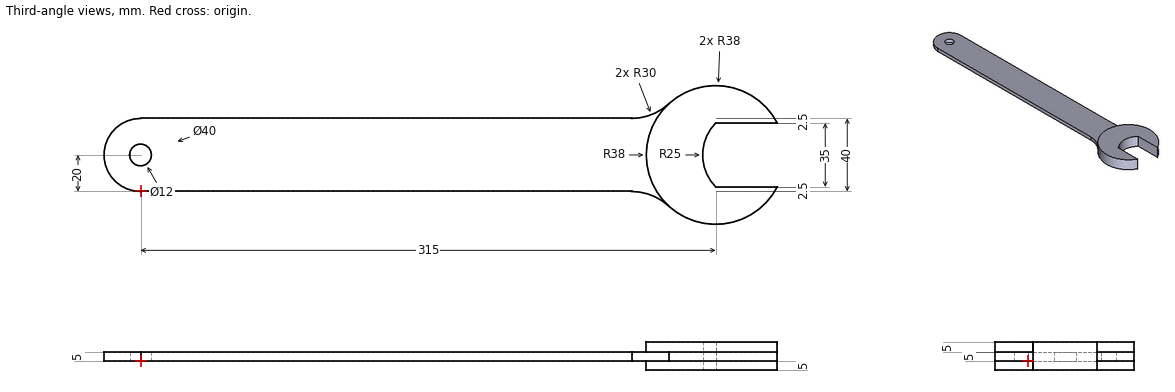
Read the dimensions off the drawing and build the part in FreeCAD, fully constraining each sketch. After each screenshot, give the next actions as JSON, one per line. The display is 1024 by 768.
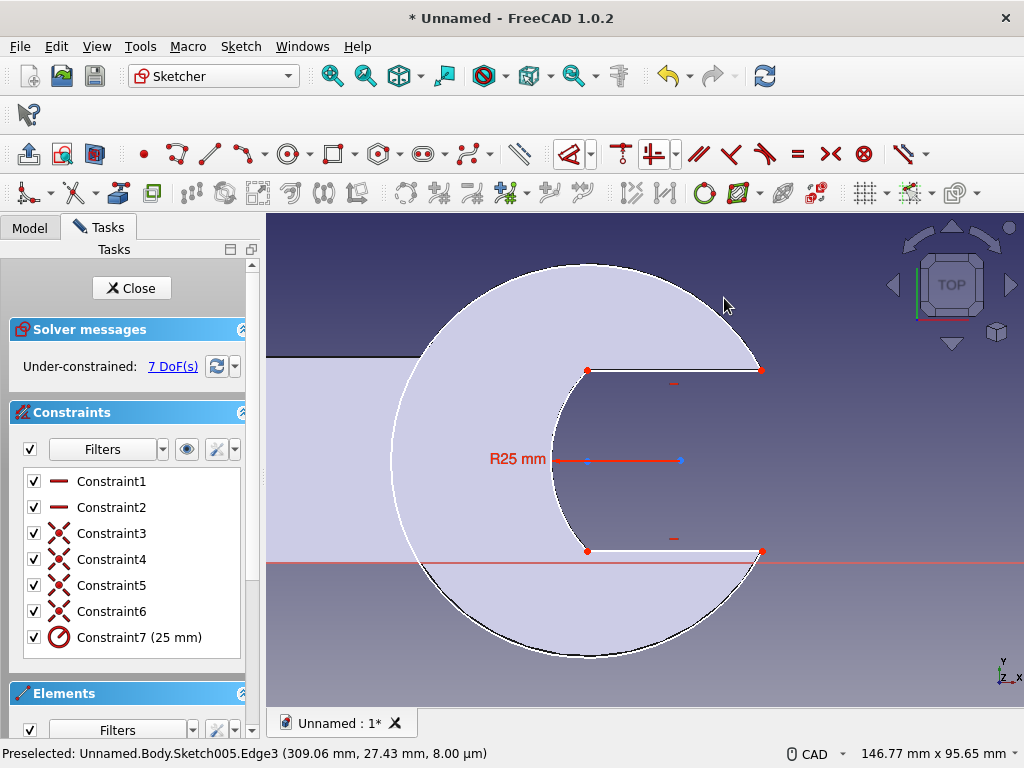
{"action": "left_click", "coordinate": [492, 290]}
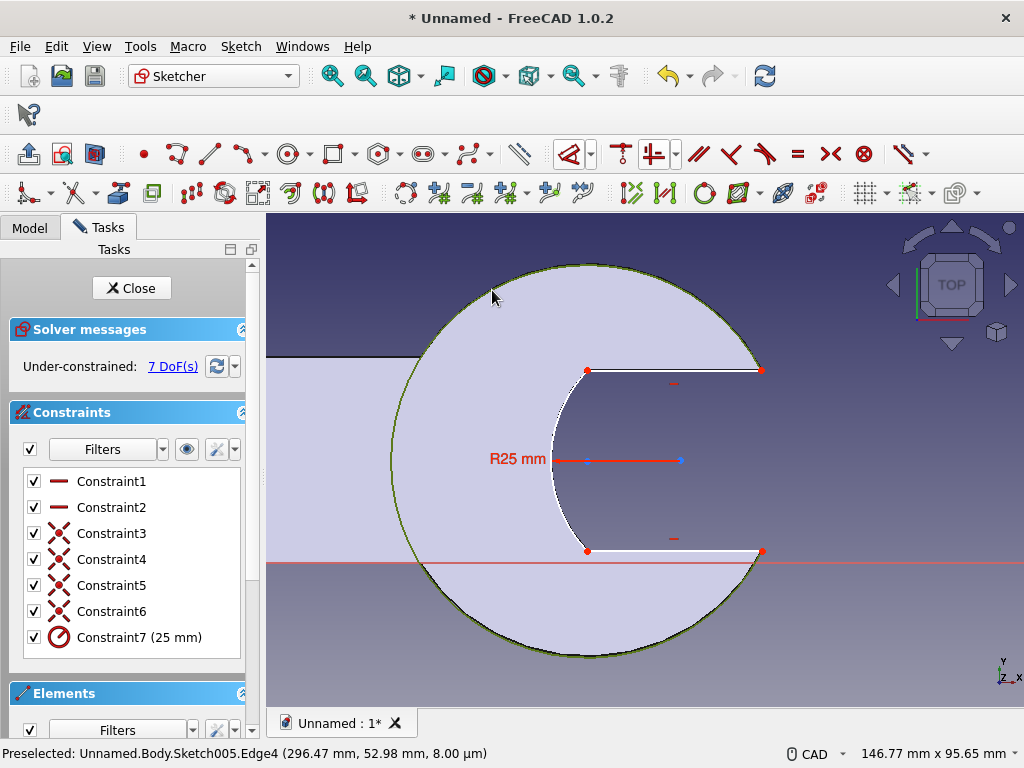
{"action": "left_click", "coordinate": [590, 154]}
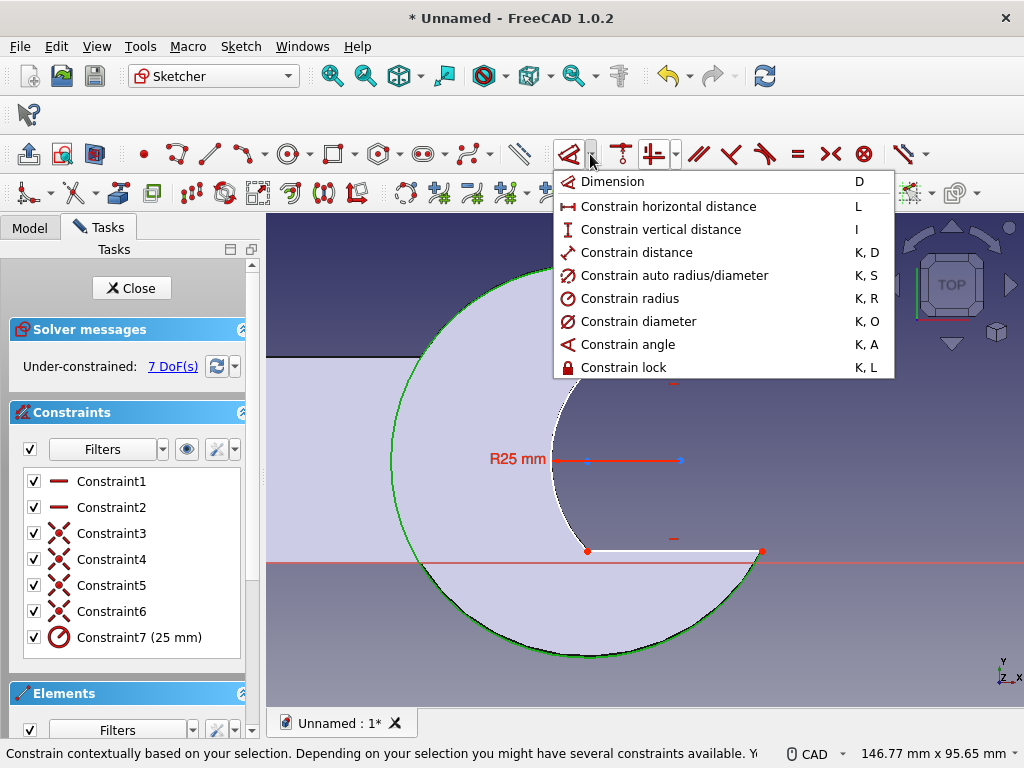
{"action": "left_click", "coordinate": [724, 298]}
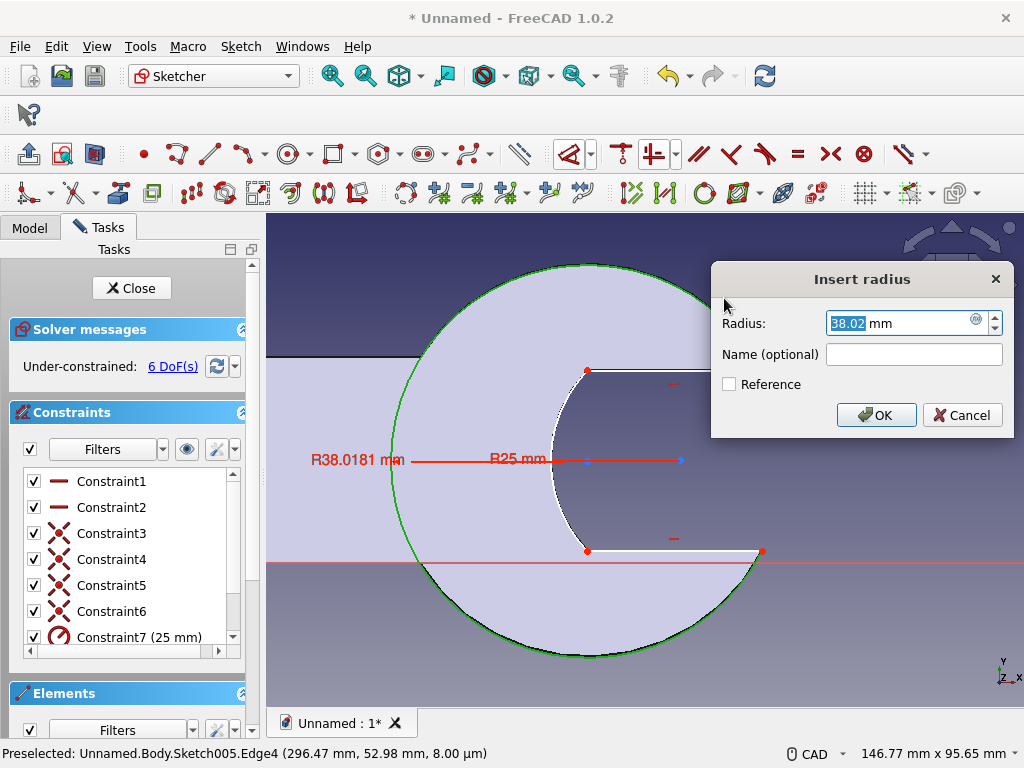
{"action": "type", "text": "38"}
{"action": "key", "text": "Return"}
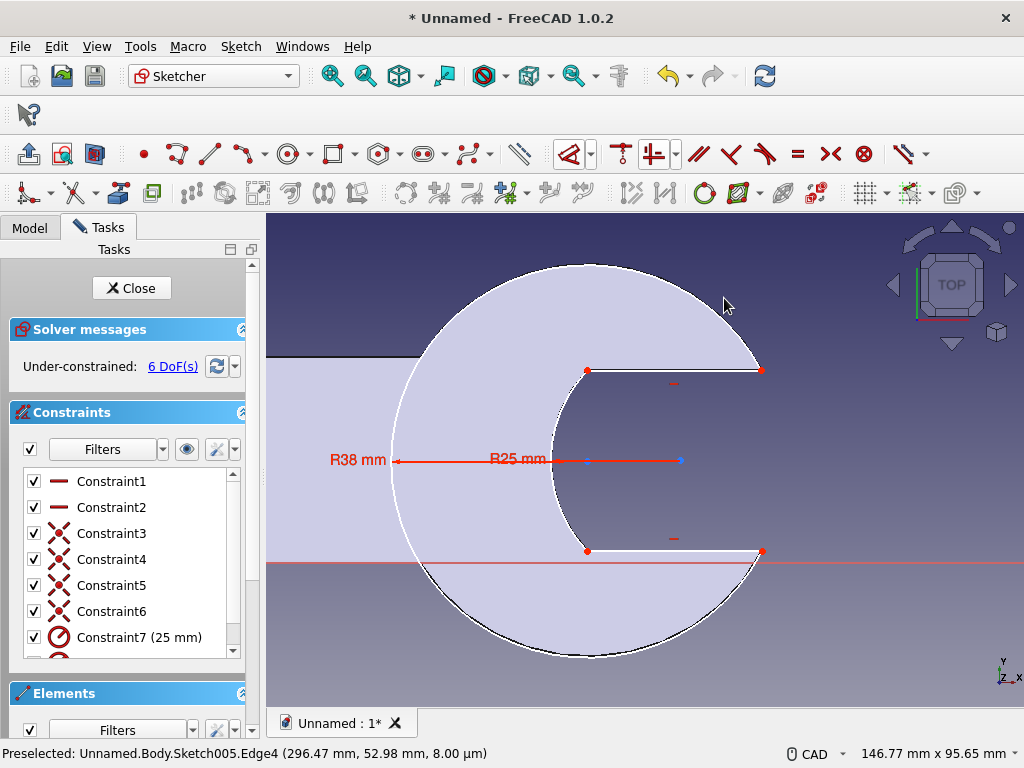
{"action": "left_click", "coordinate": [680, 461]}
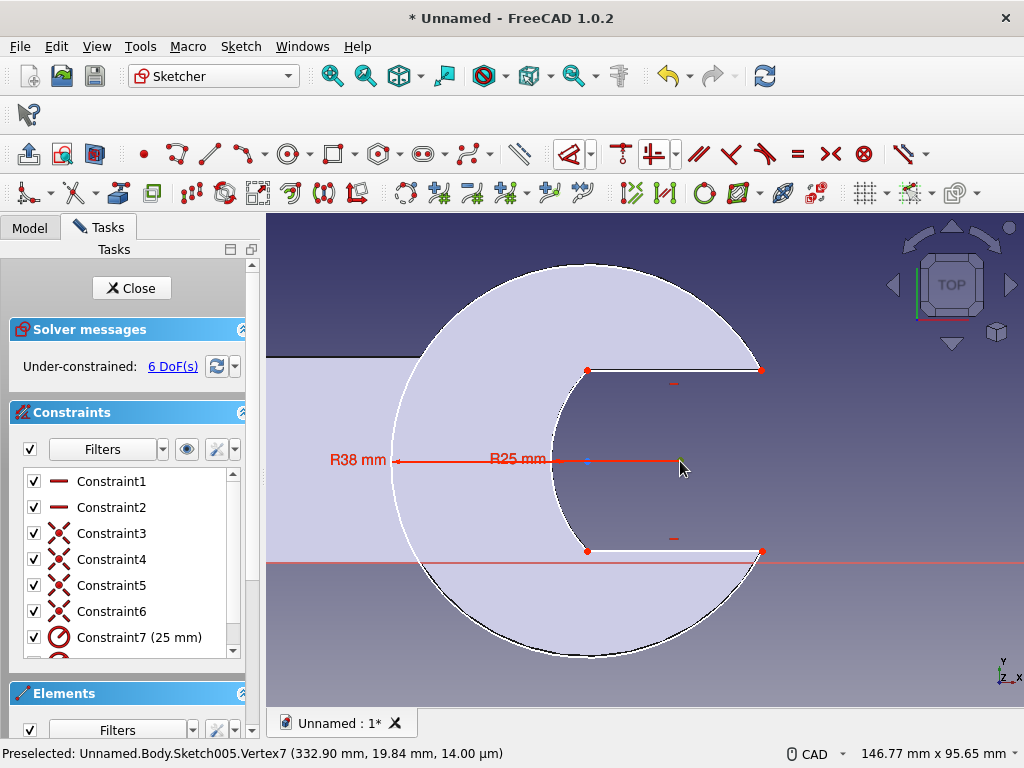
{"action": "left_click", "coordinate": [590, 154]}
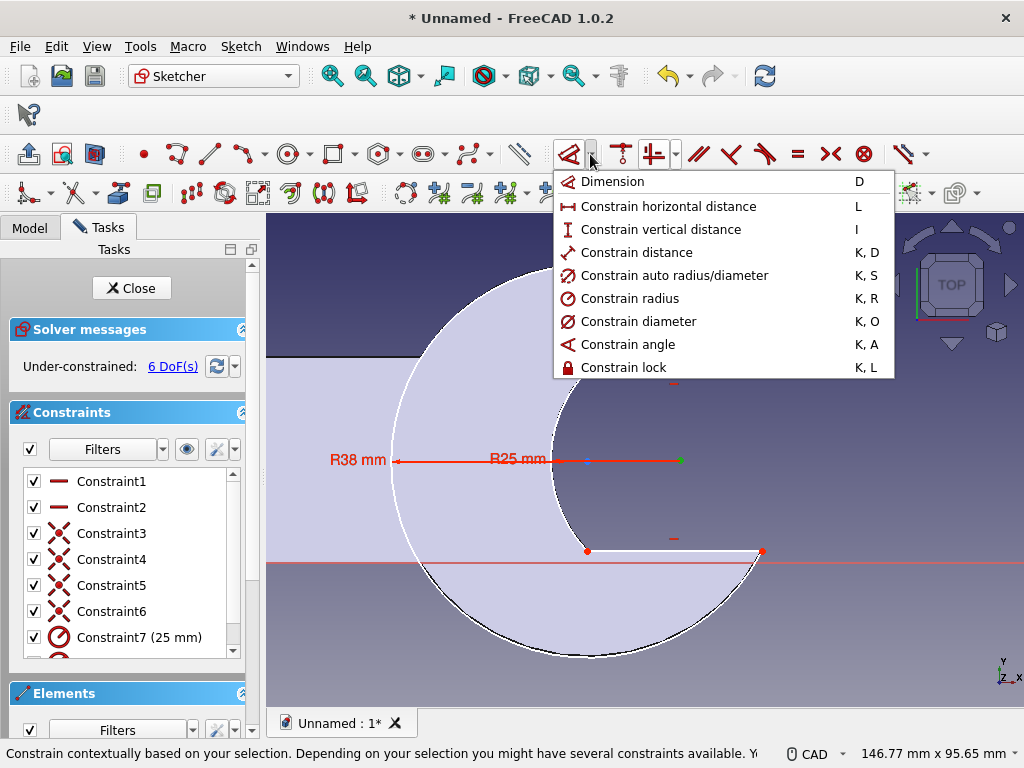
{"action": "left_click", "coordinate": [724, 230]}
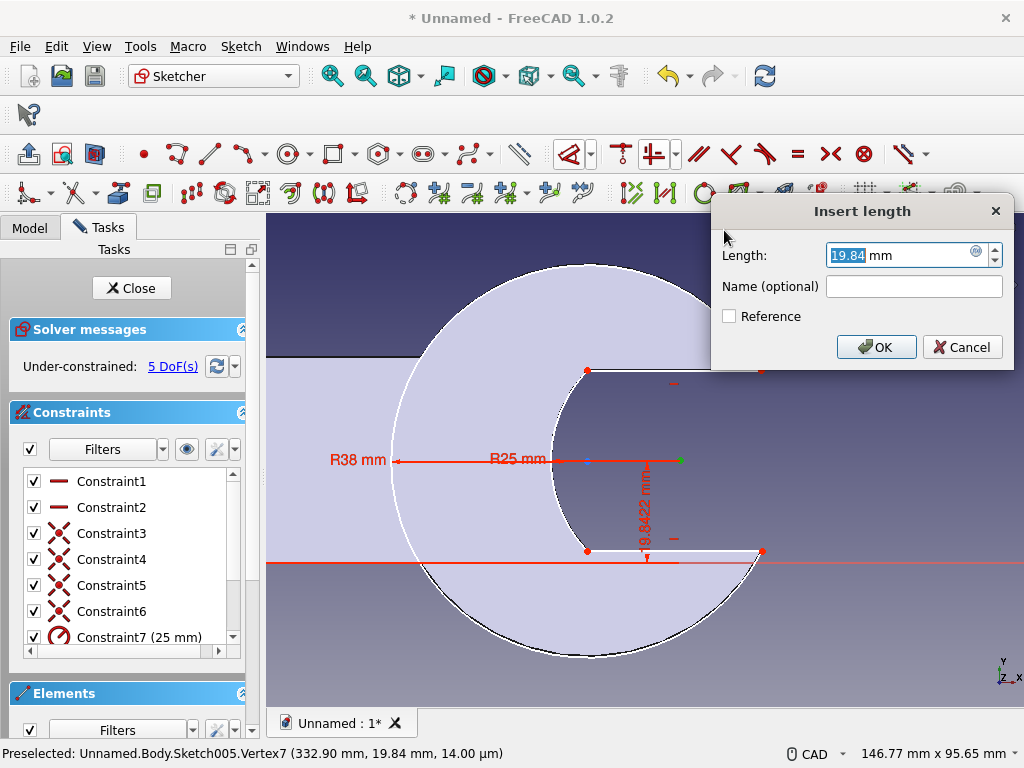
{"action": "type", "text": "20"}
{"action": "key", "text": "Return"}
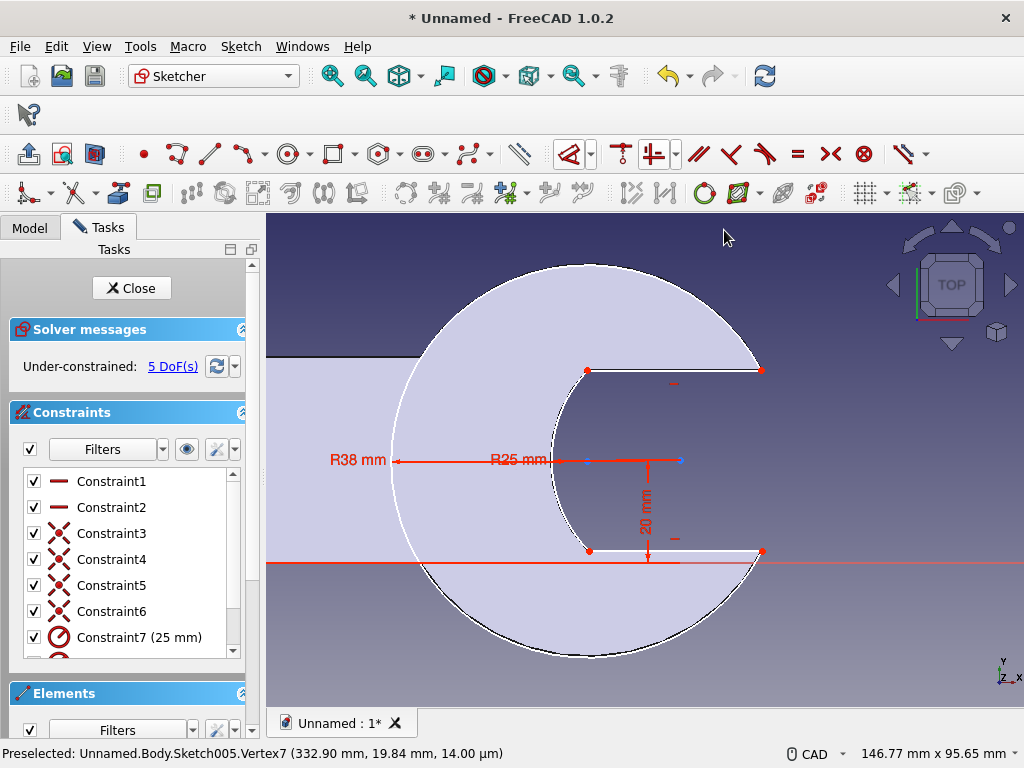
{"action": "left_click", "coordinate": [587, 461]}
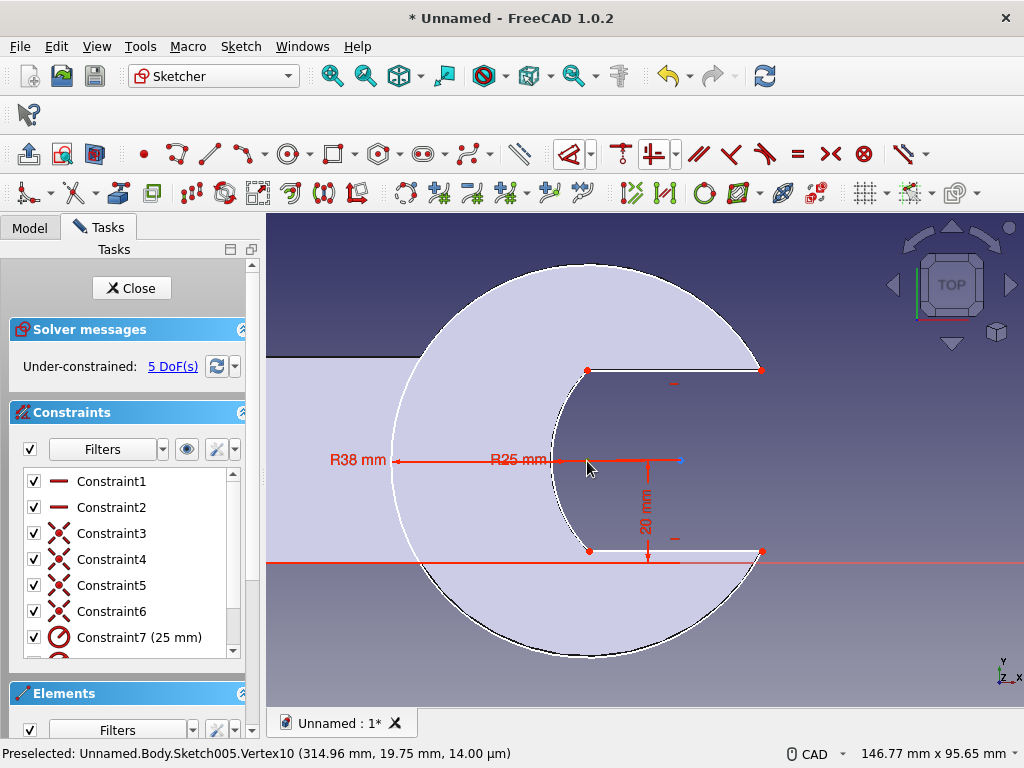
{"action": "left_click", "coordinate": [590, 154]}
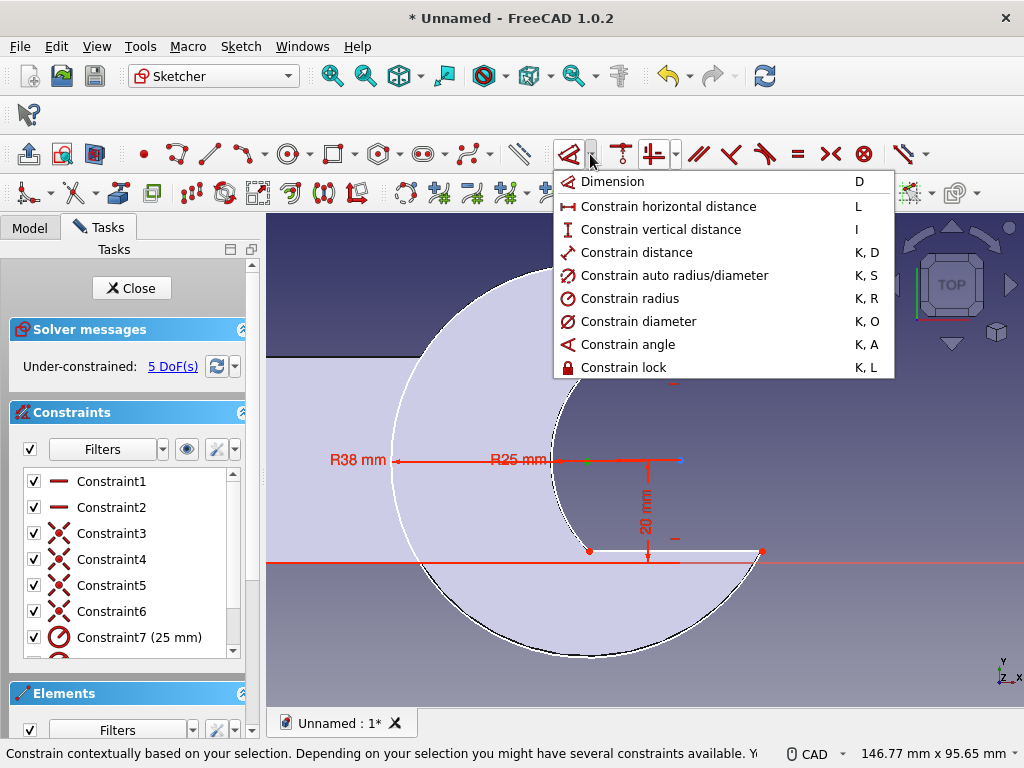
{"action": "left_click", "coordinate": [724, 230]}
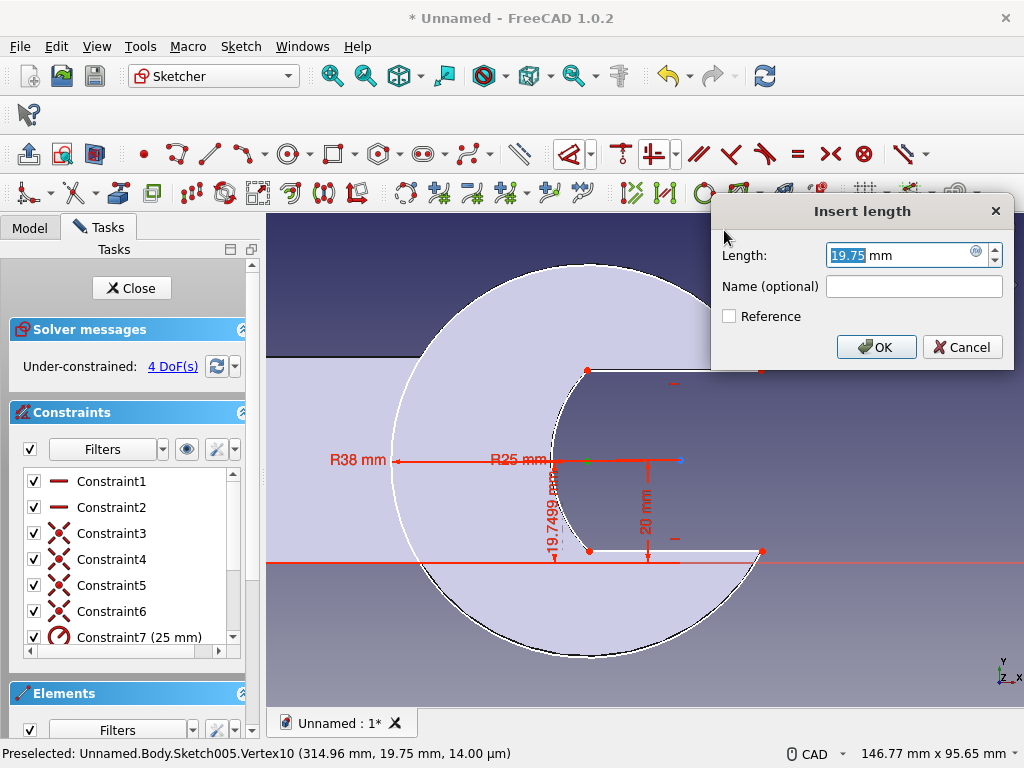
{"action": "type", "text": "20"}
{"action": "key", "text": "Return"}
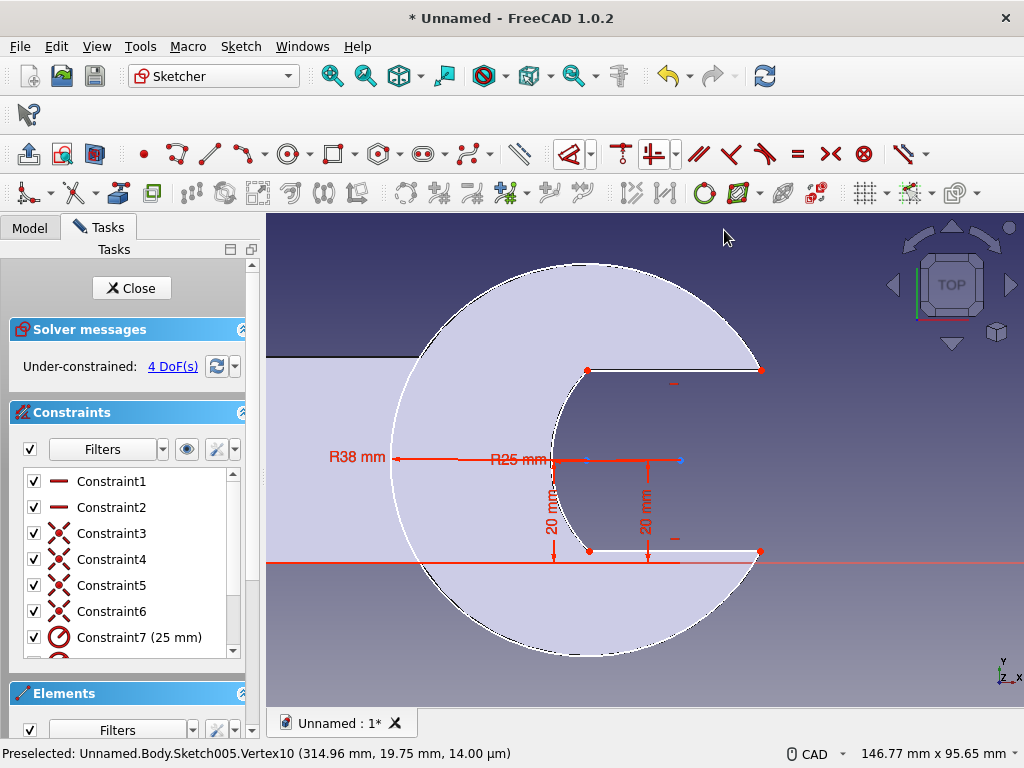
{"action": "left_click", "coordinate": [588, 371]}